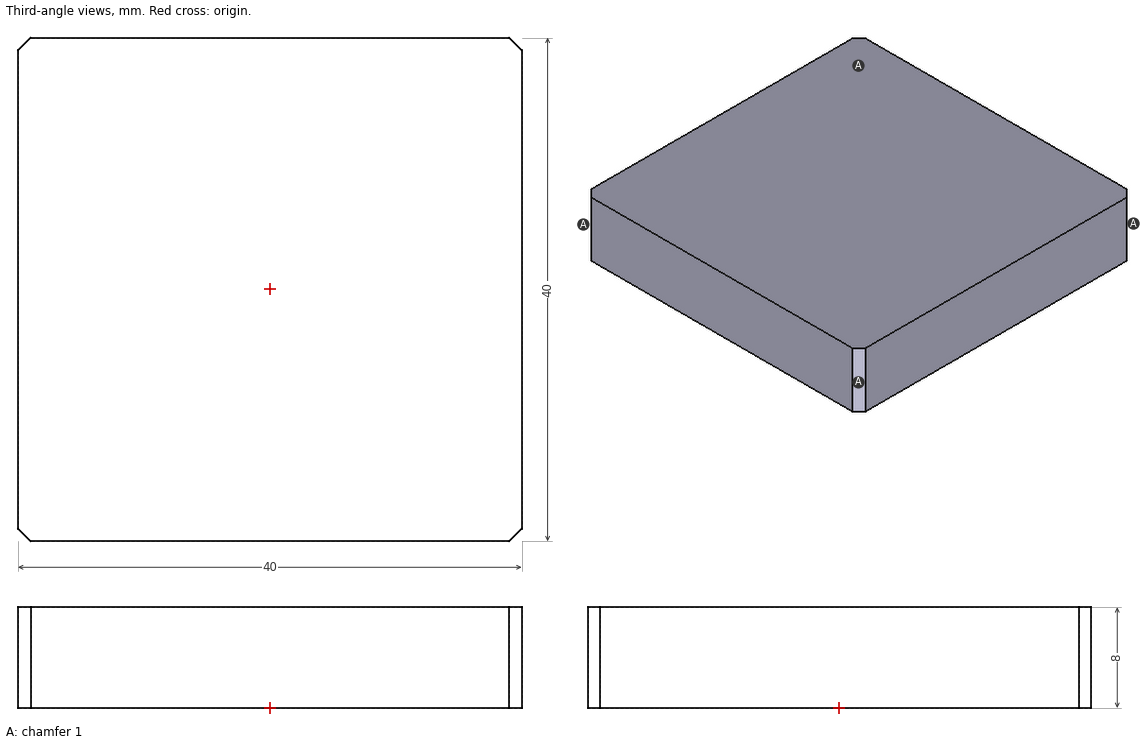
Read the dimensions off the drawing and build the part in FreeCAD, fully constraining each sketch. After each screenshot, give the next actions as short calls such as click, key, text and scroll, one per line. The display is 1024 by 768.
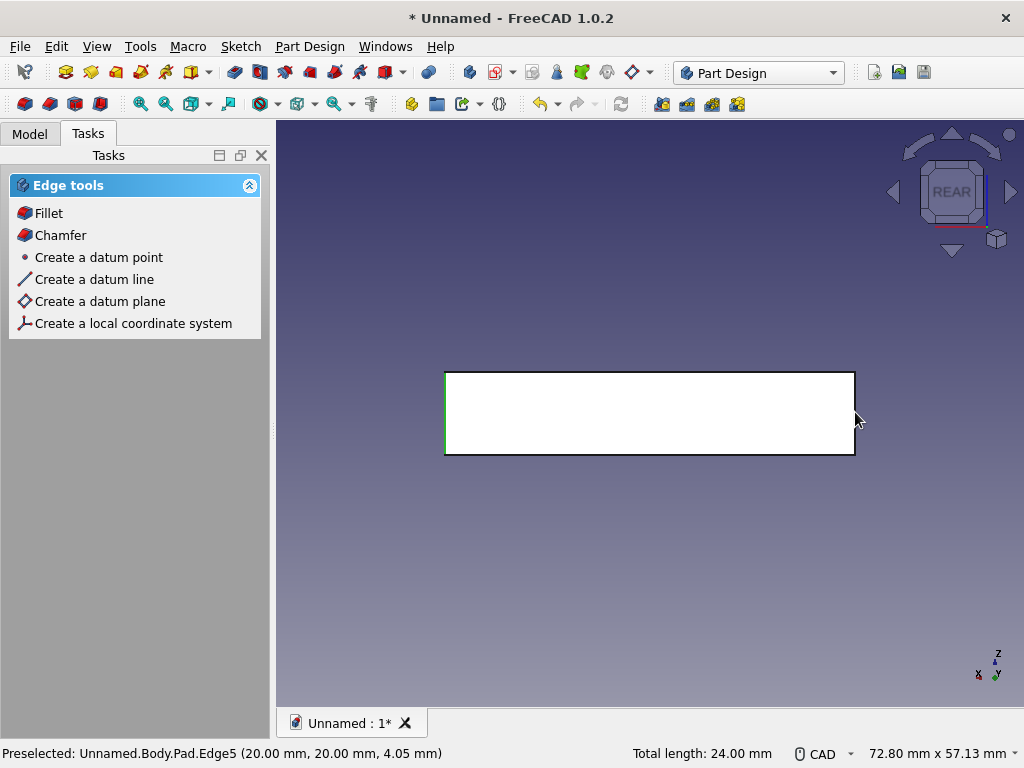
click(855, 412, ctrl)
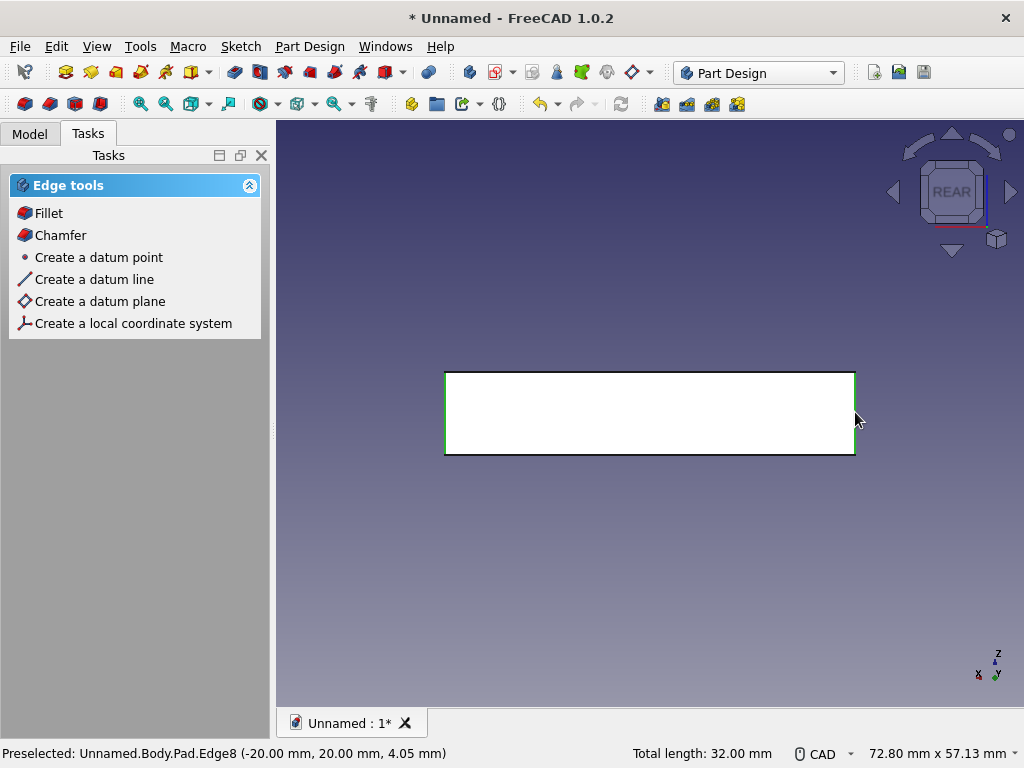
click(50, 104)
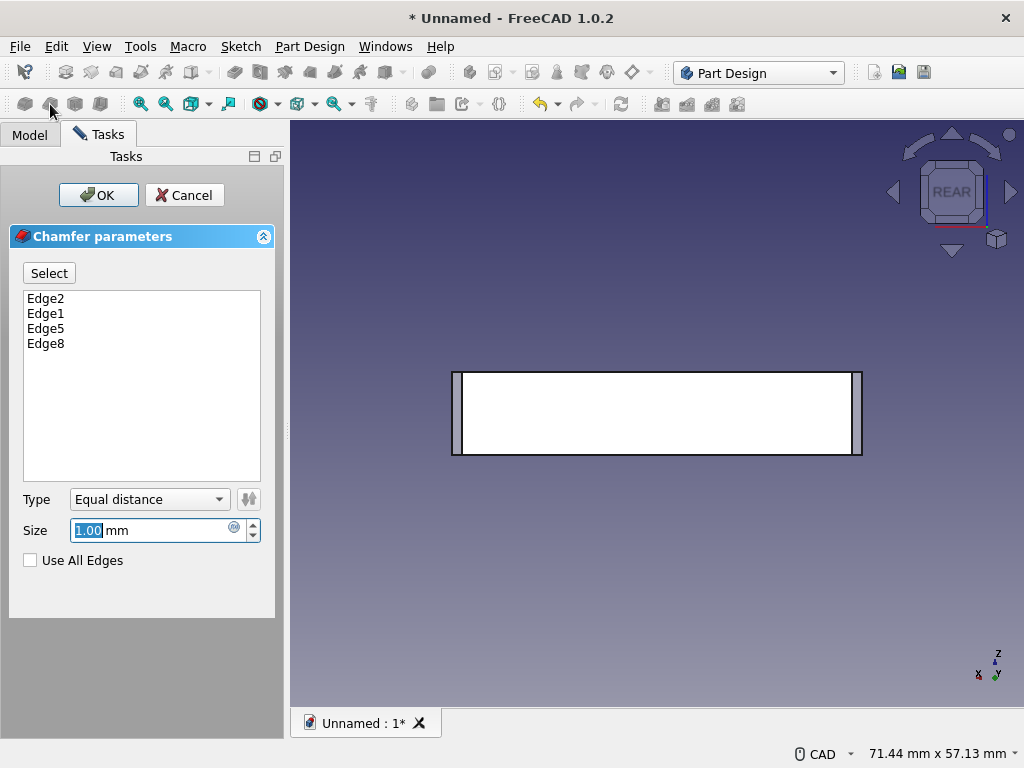
text(1)
key(Tab)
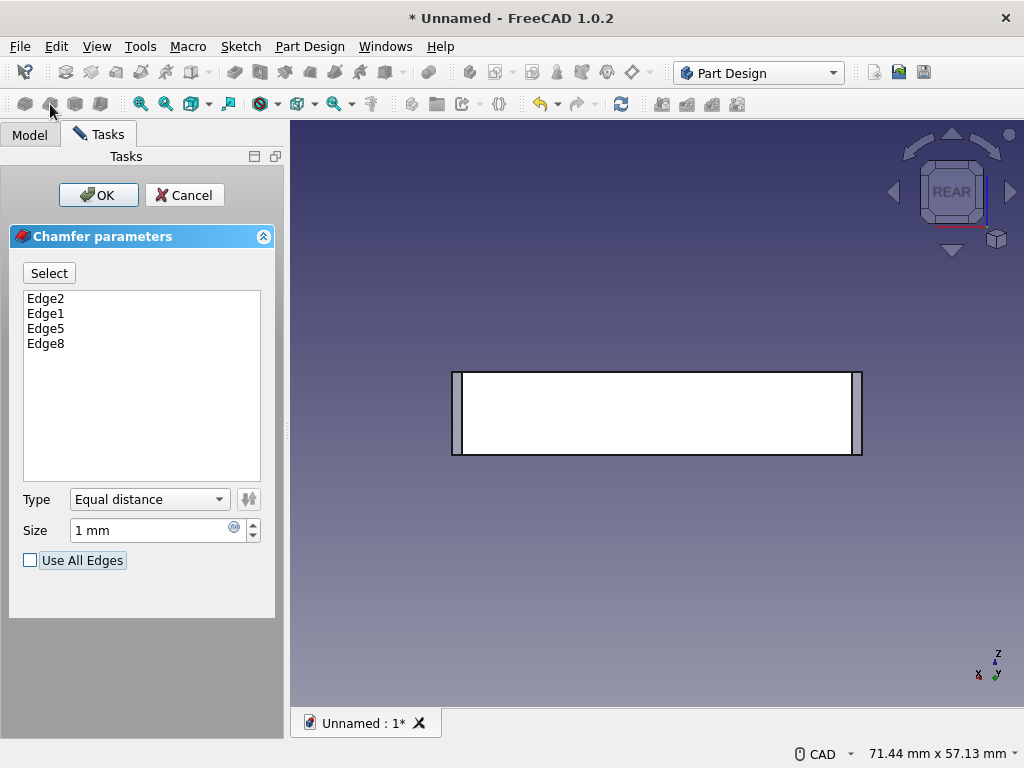
click(99, 195)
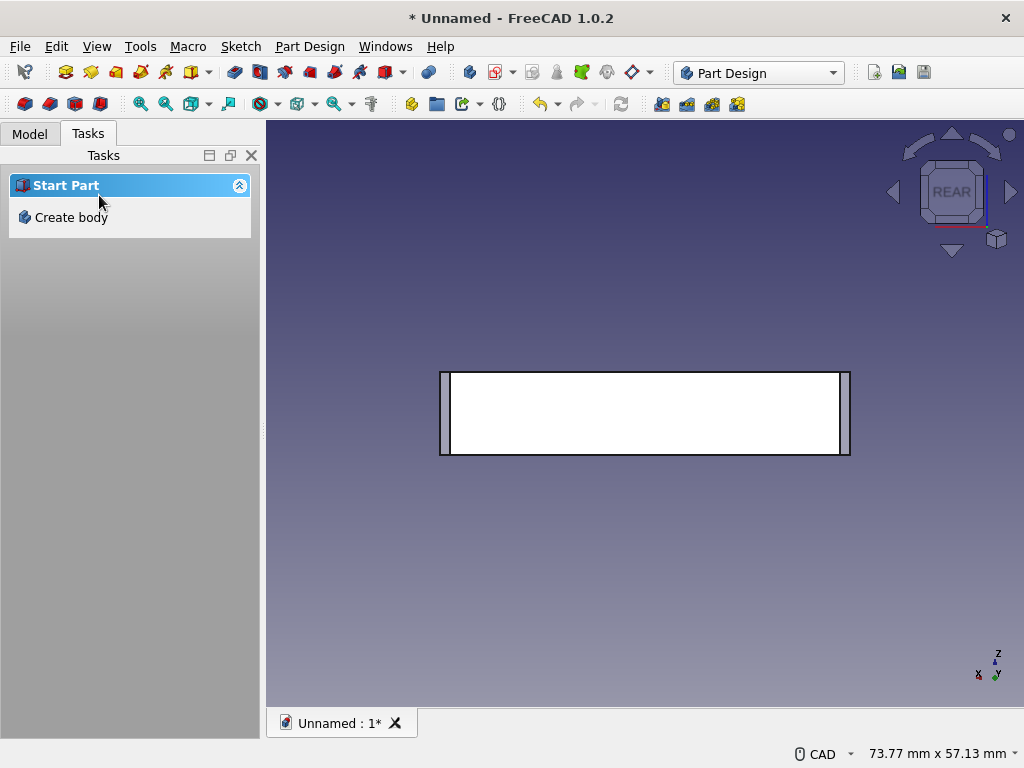
key(0)